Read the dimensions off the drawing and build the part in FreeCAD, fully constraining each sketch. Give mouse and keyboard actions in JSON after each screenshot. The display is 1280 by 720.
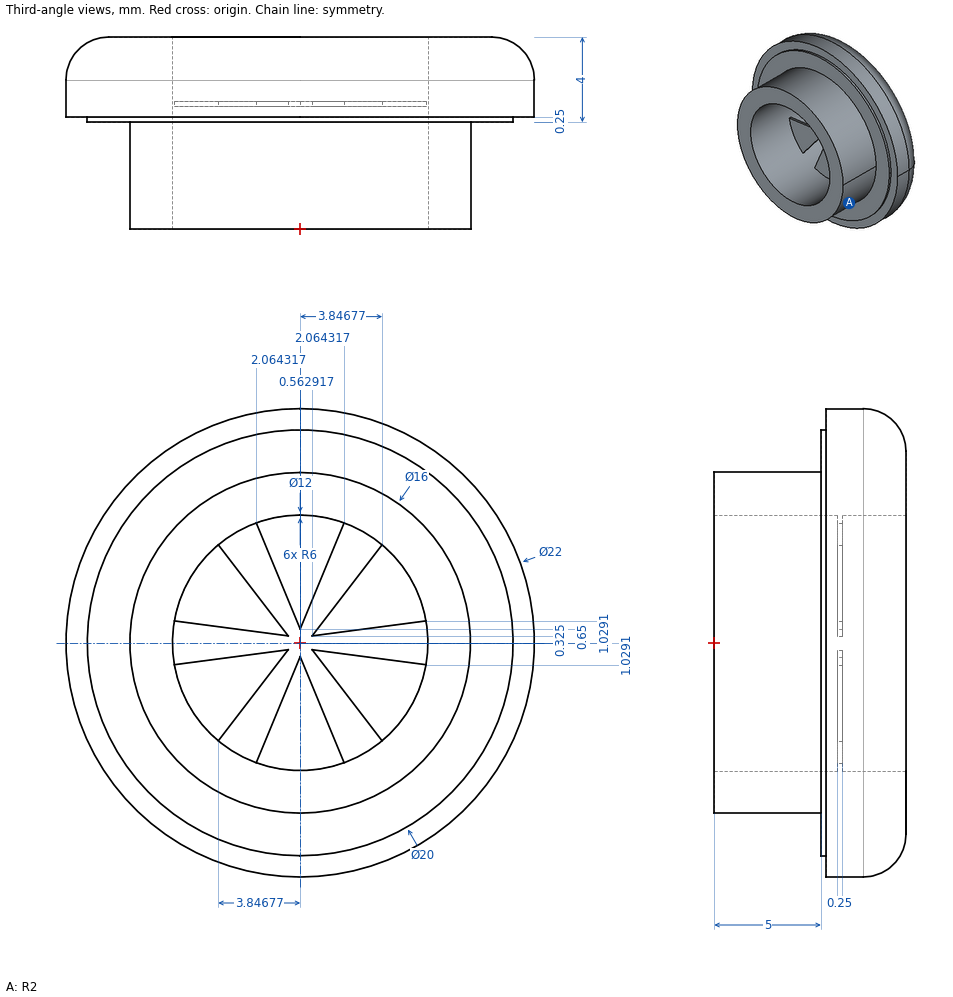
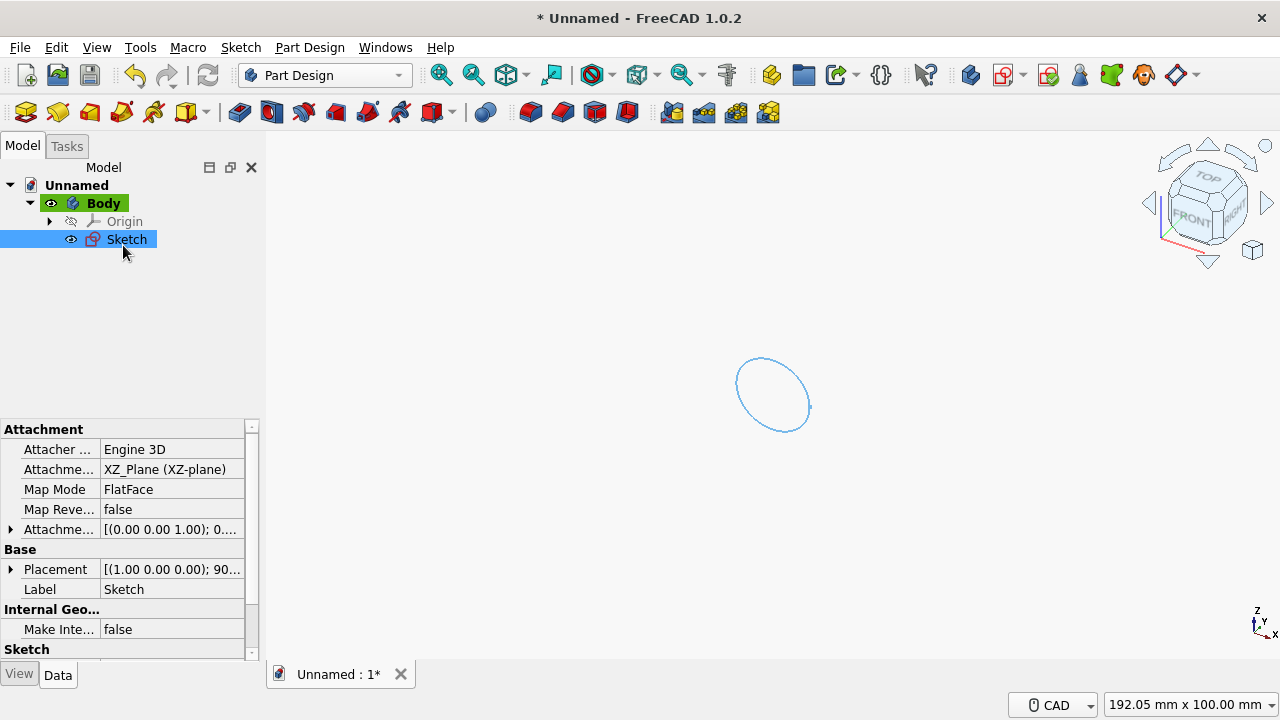
{"action": "left_click", "coordinate": [26, 112]}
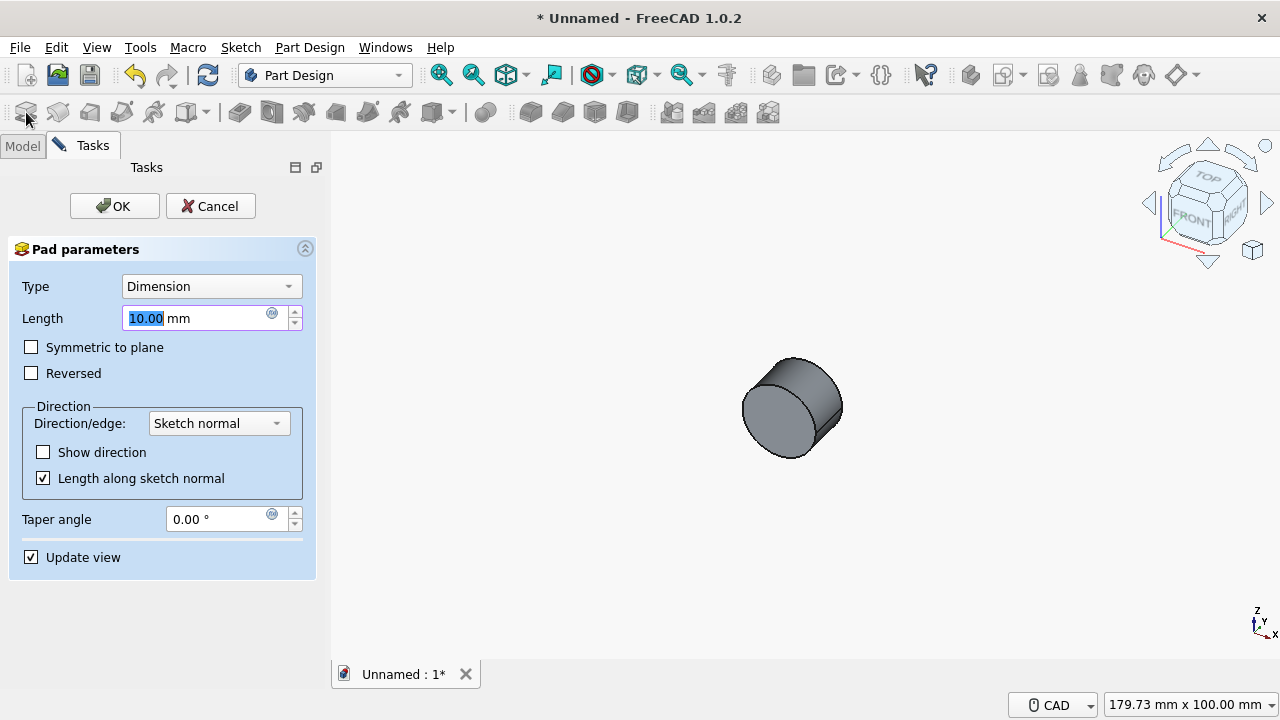
{"action": "type", "text": "5"}
{"action": "key", "text": "Tab"}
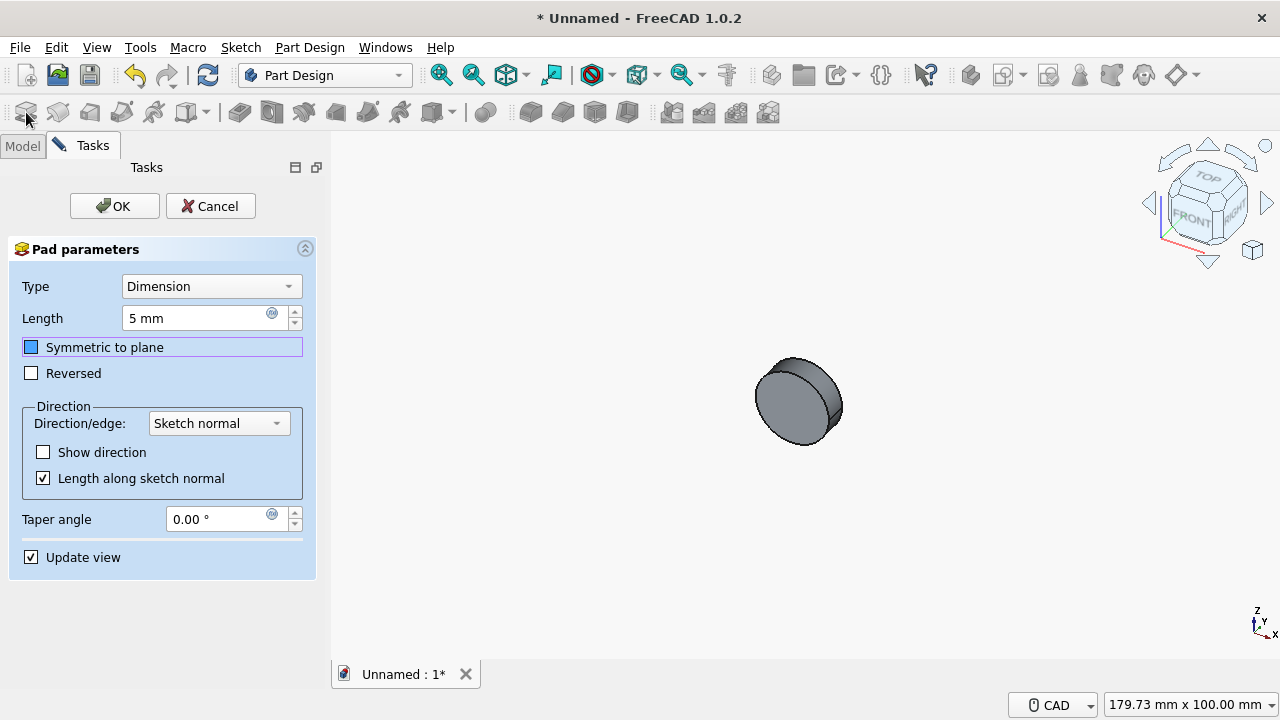
{"action": "left_click", "coordinate": [30, 373]}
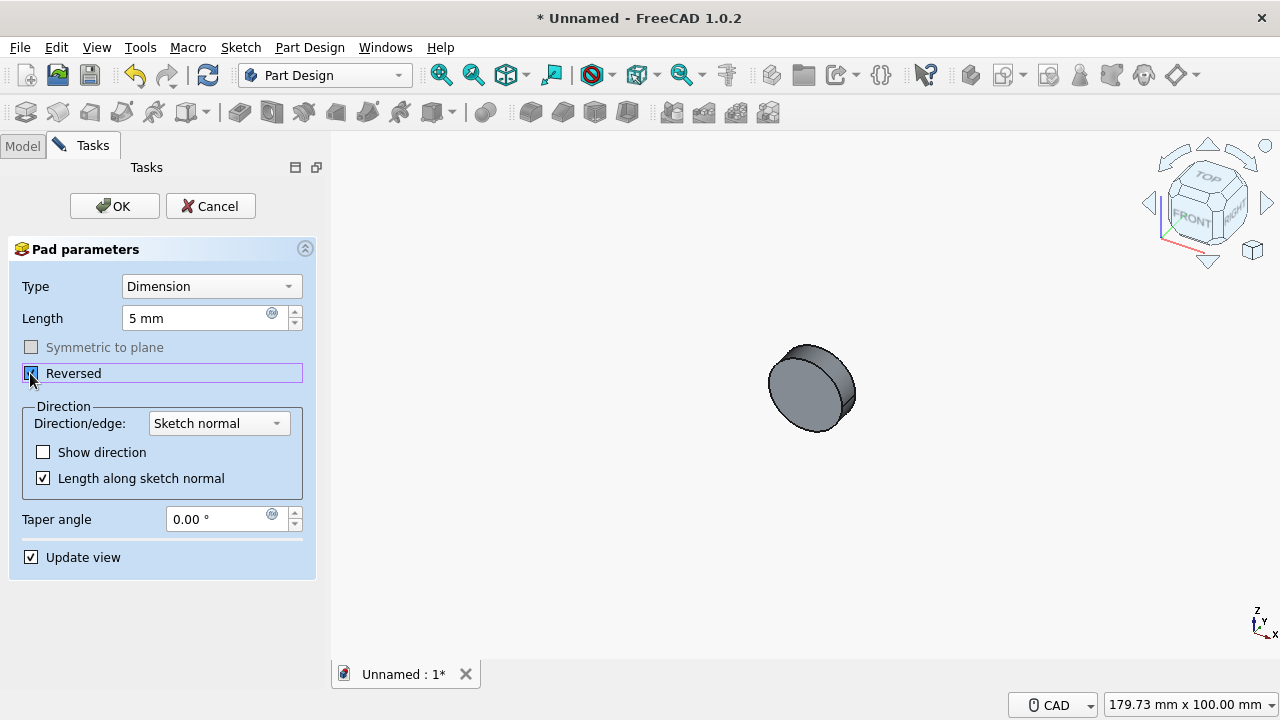
{"action": "left_click", "coordinate": [115, 206]}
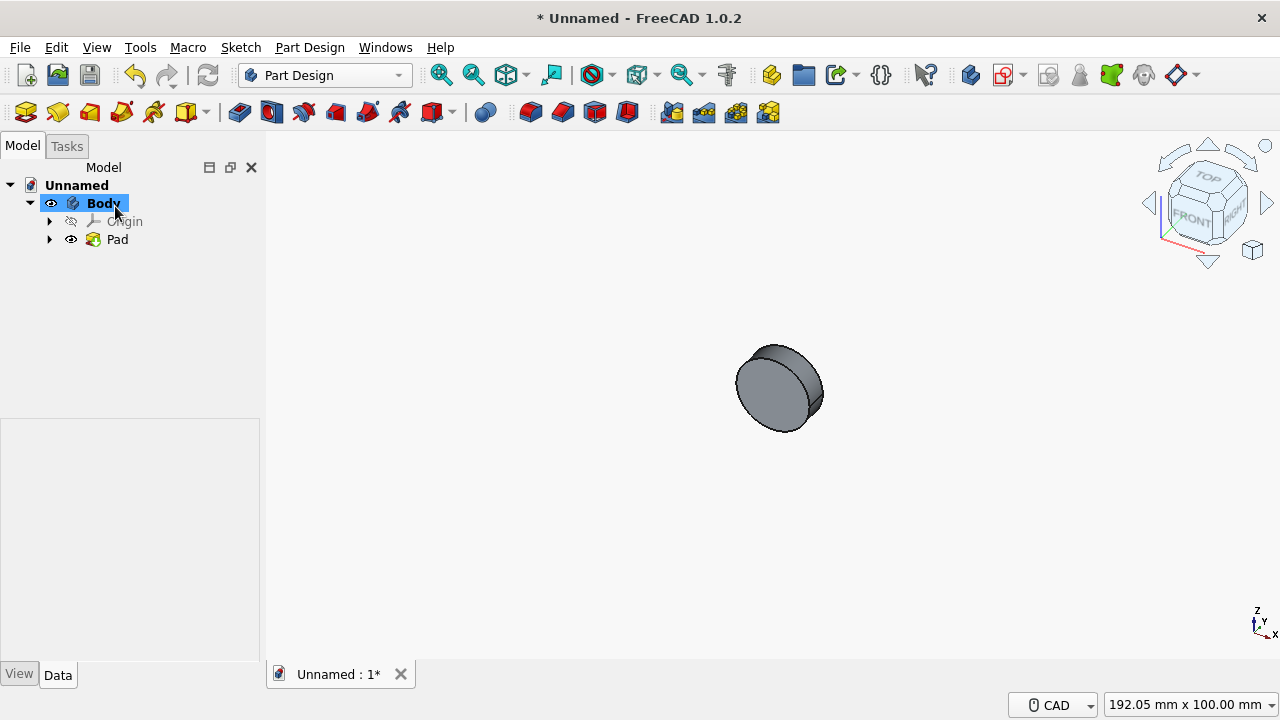
{"action": "key", "text": "v f"}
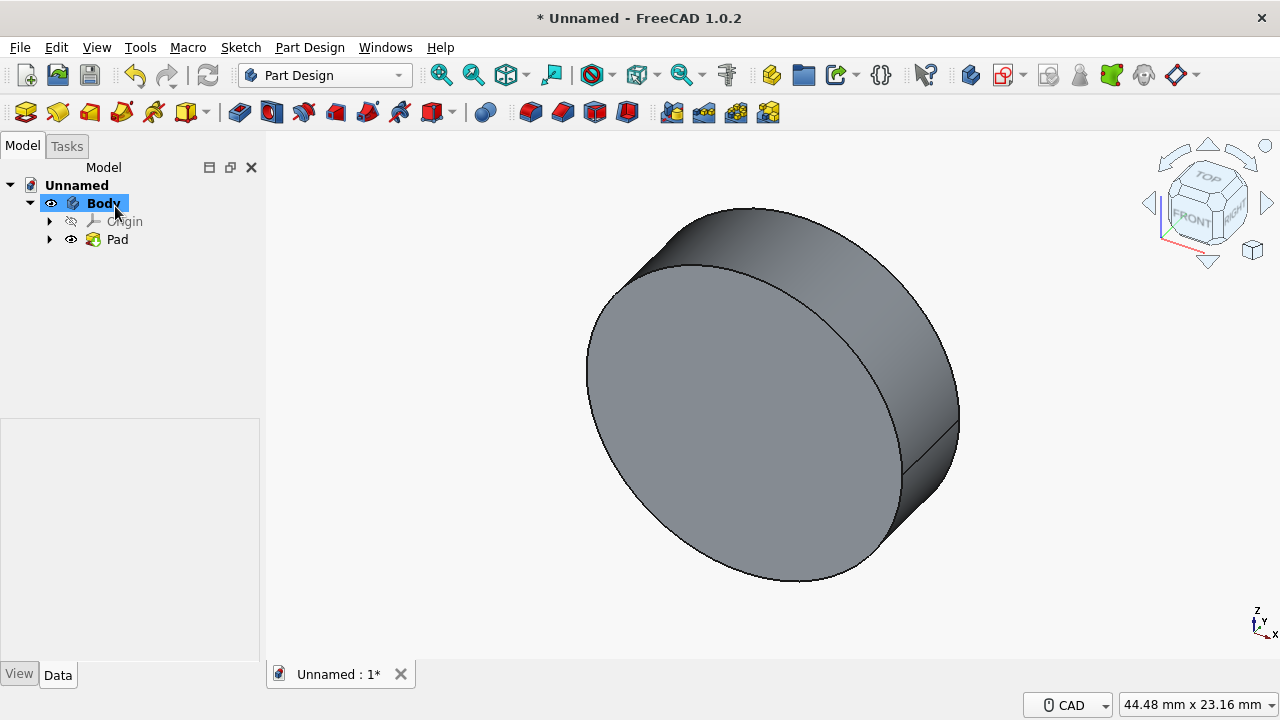
{"action": "key", "text": "4"}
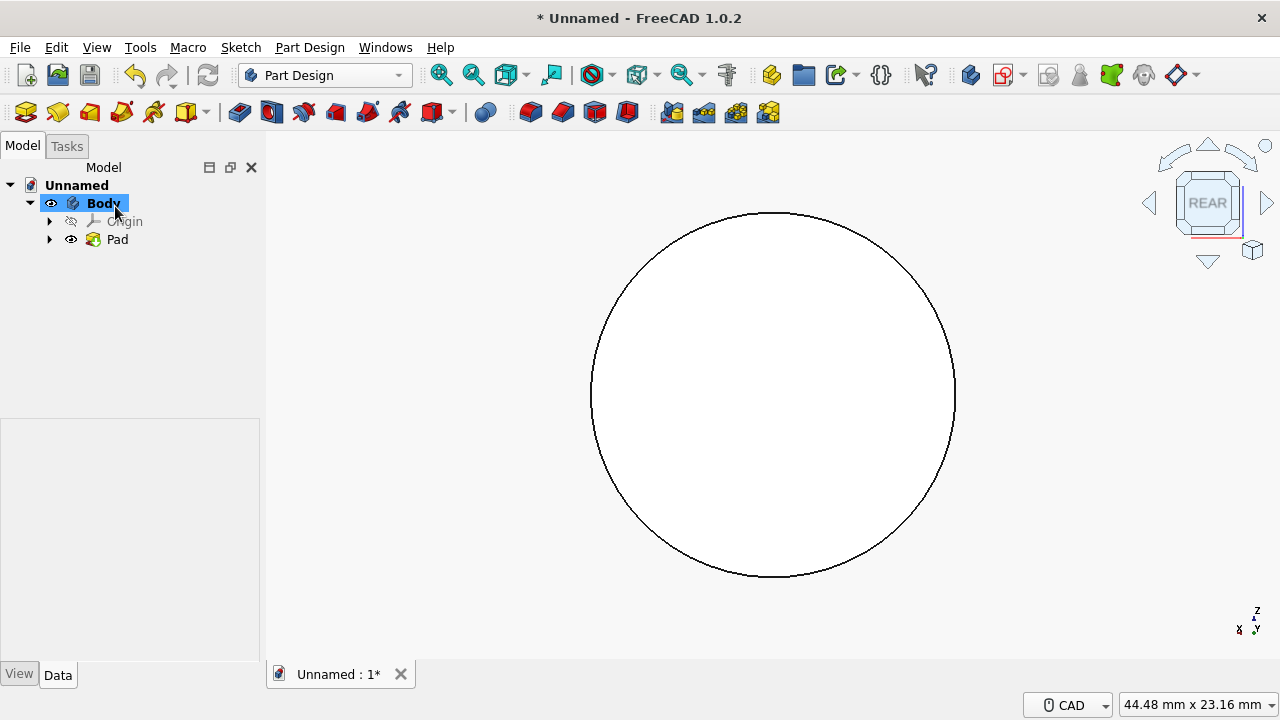
{"action": "left_click", "coordinate": [773, 394]}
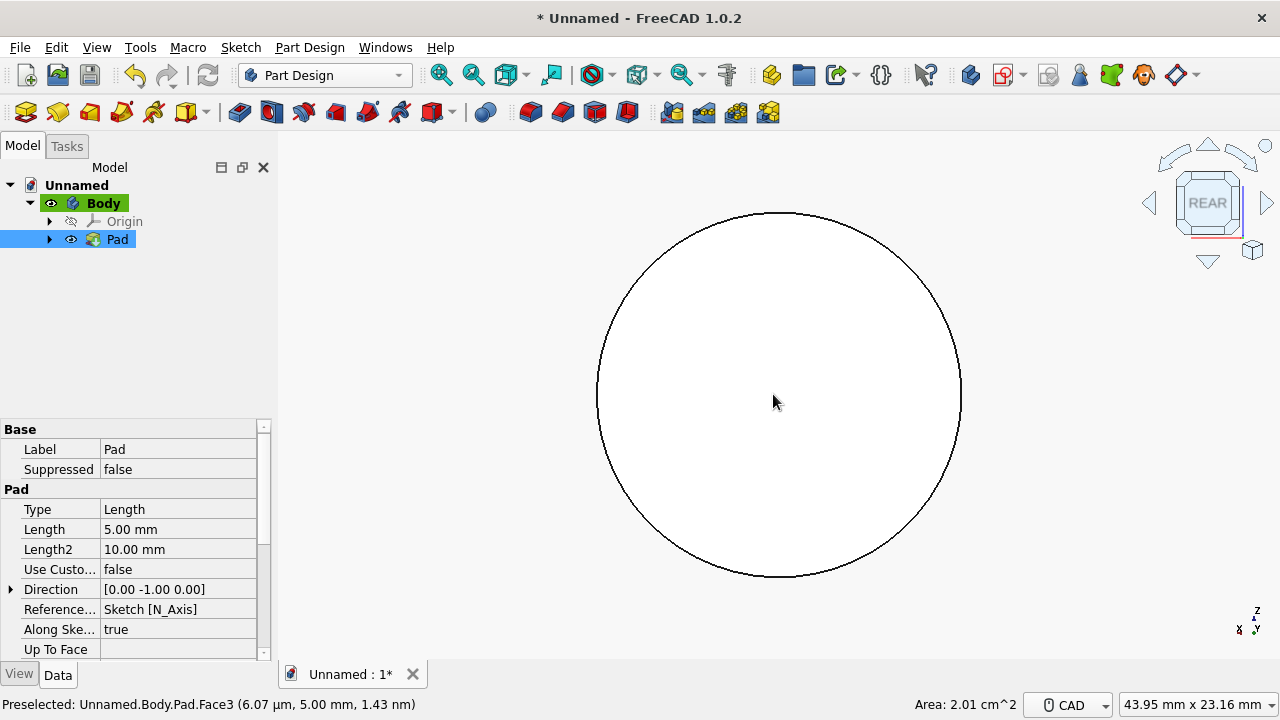
{"action": "left_click", "coordinate": [1004, 76]}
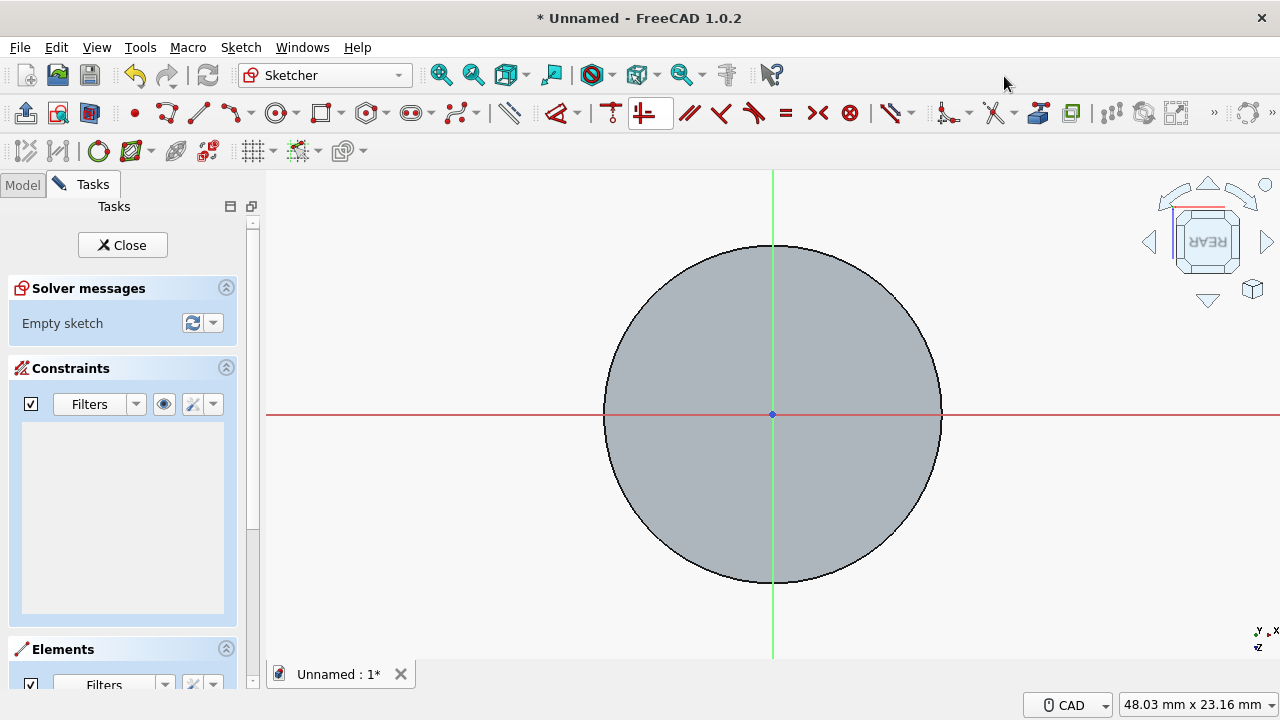
{"action": "scroll", "coordinate": [565, 415], "scroll_direction": "down", "scroll_amount": 2}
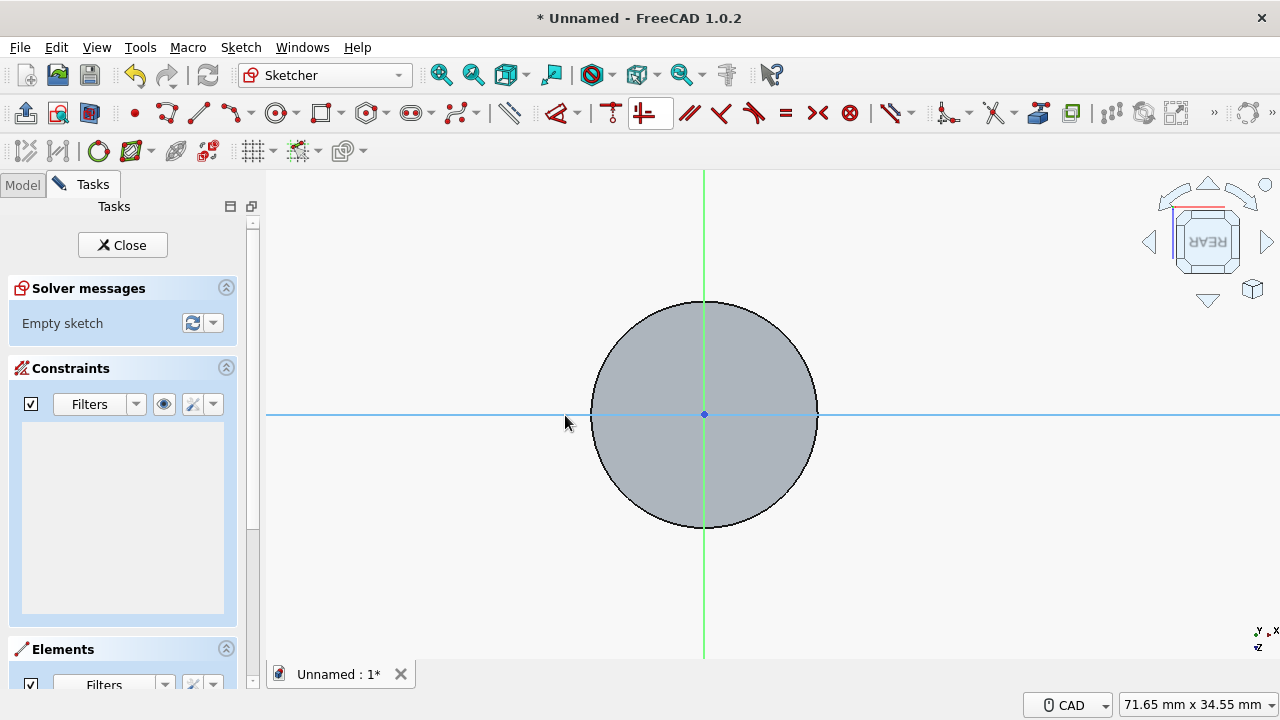
{"action": "left_click", "coordinate": [276, 114]}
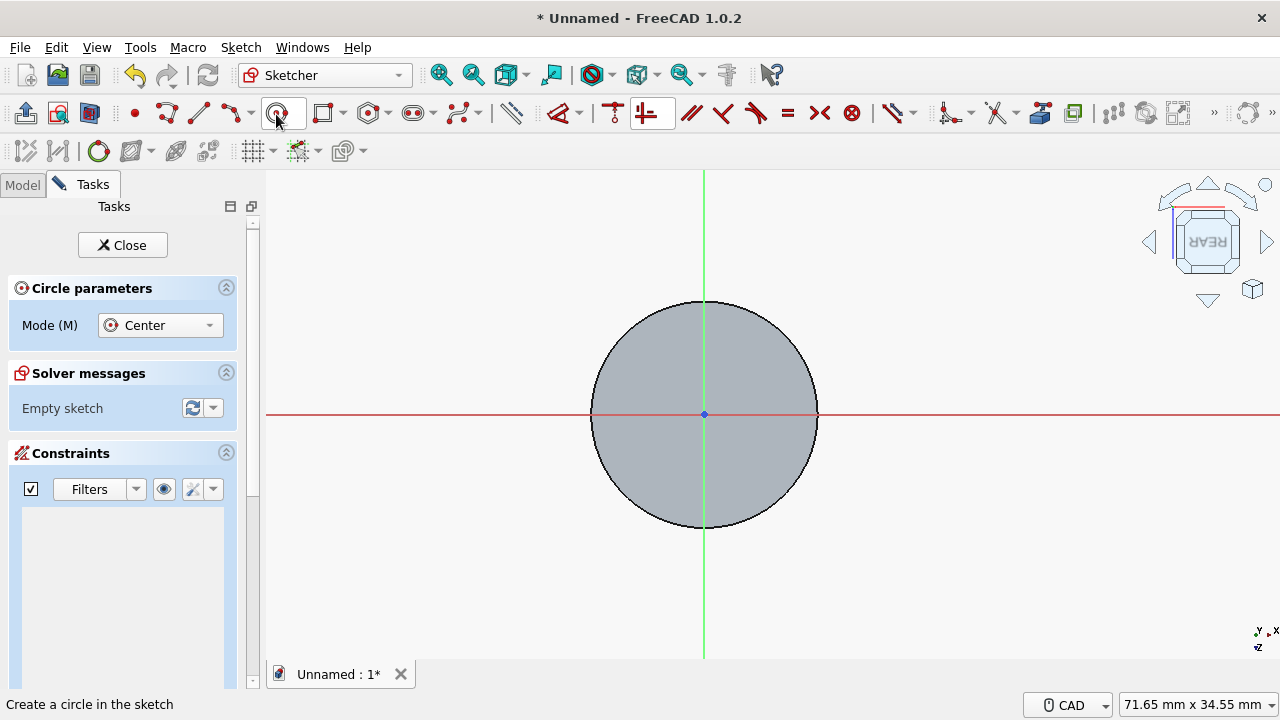
{"action": "left_click", "coordinate": [704, 415]}
{"action": "left_click", "coordinate": [815, 305]}
{"action": "key", "text": "Escape"}